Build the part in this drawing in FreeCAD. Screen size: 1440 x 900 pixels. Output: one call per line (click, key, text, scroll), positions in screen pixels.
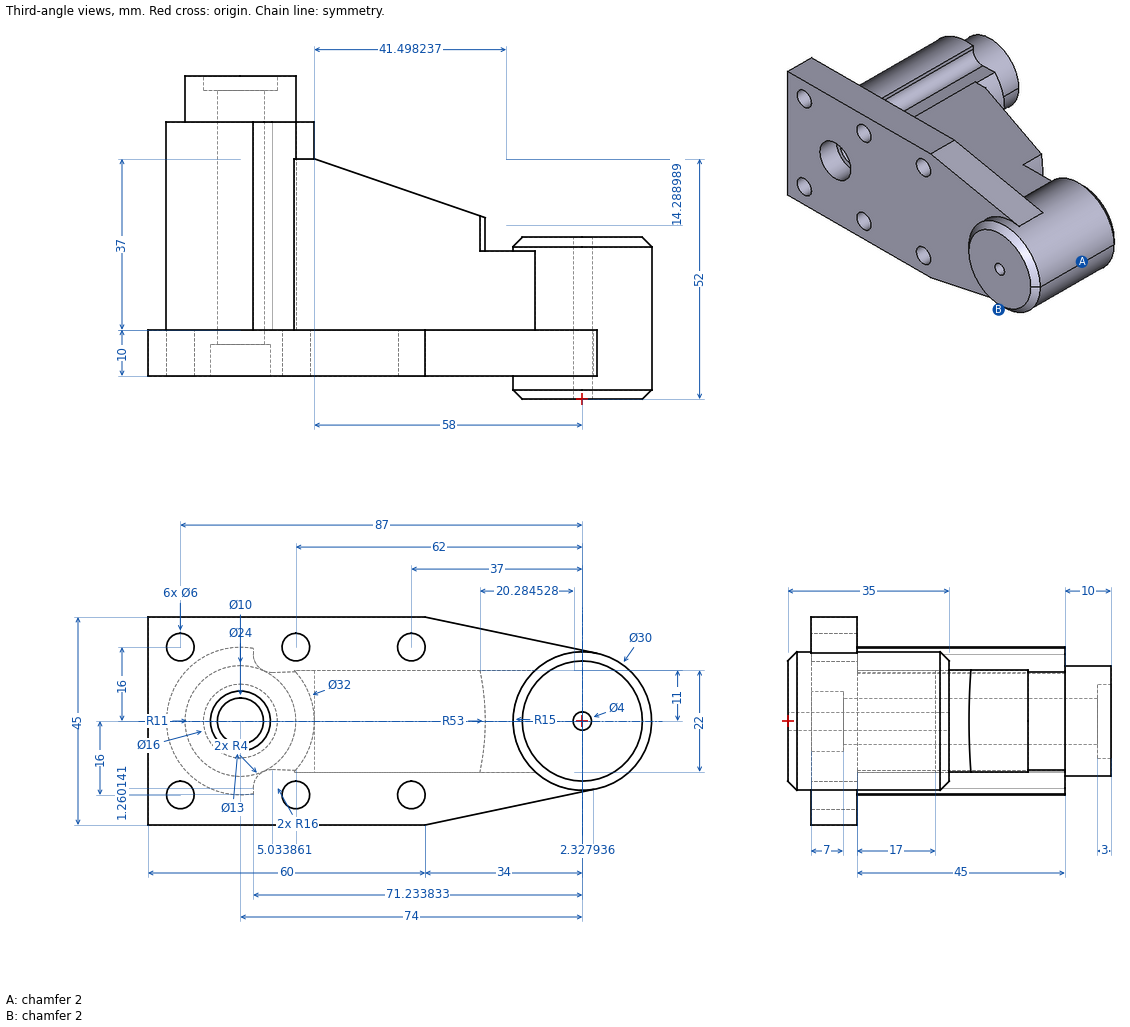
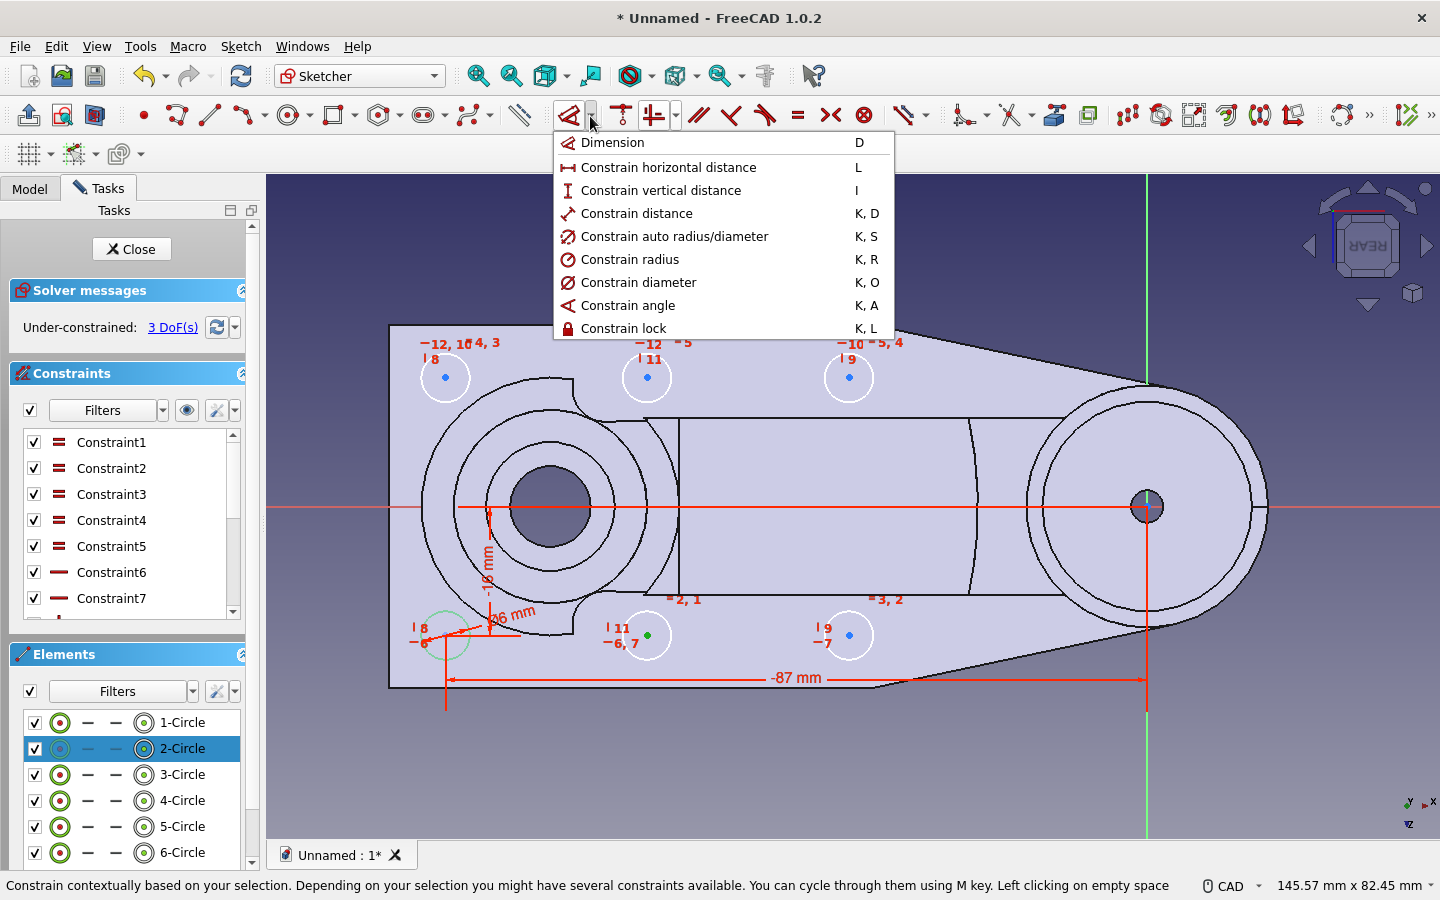
click(724, 168)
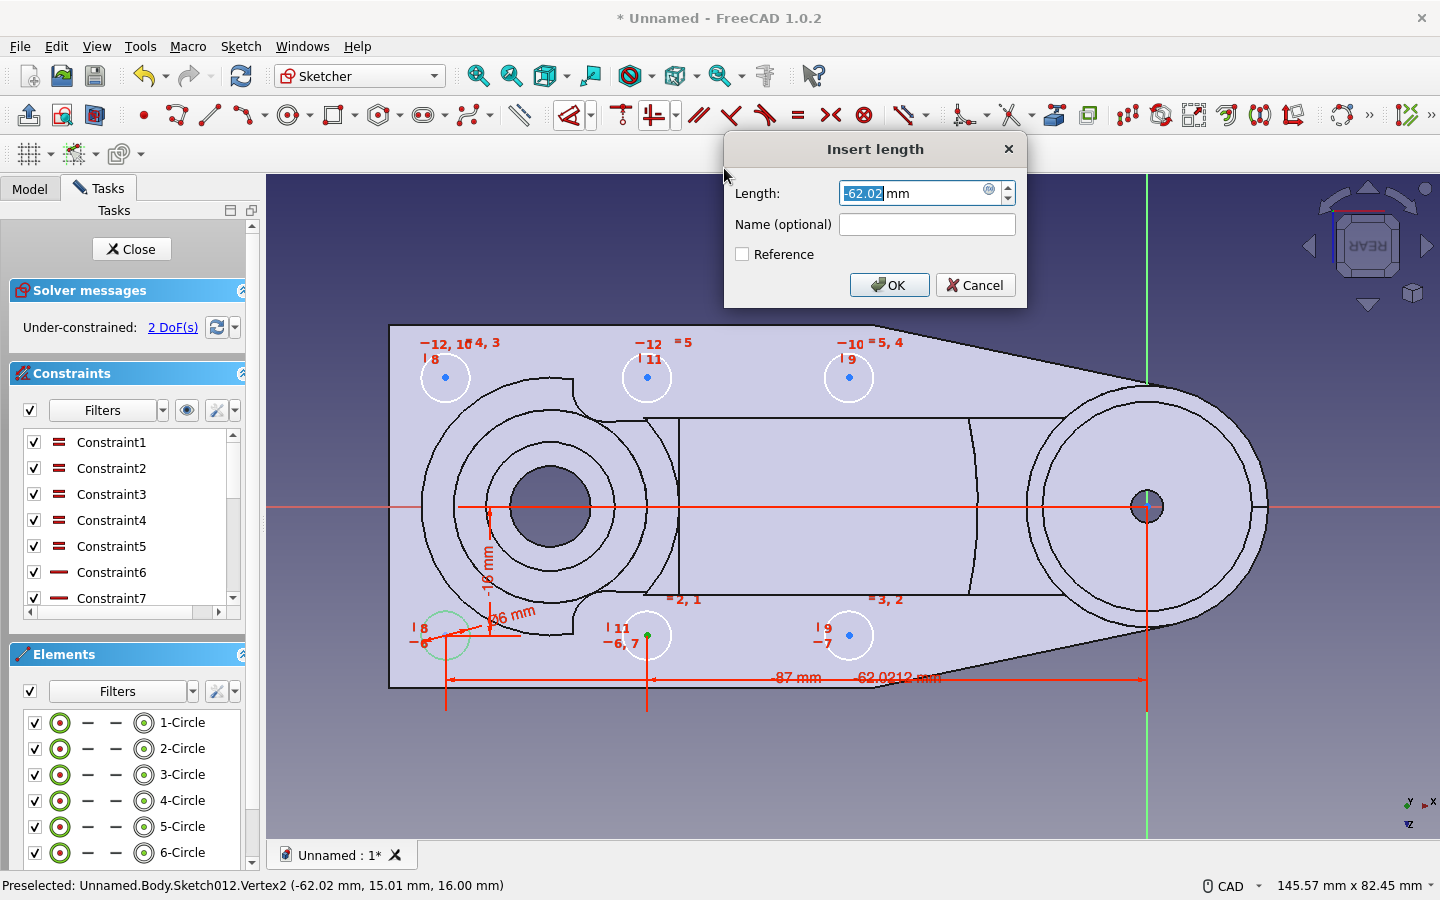
text(-62)
key(Return)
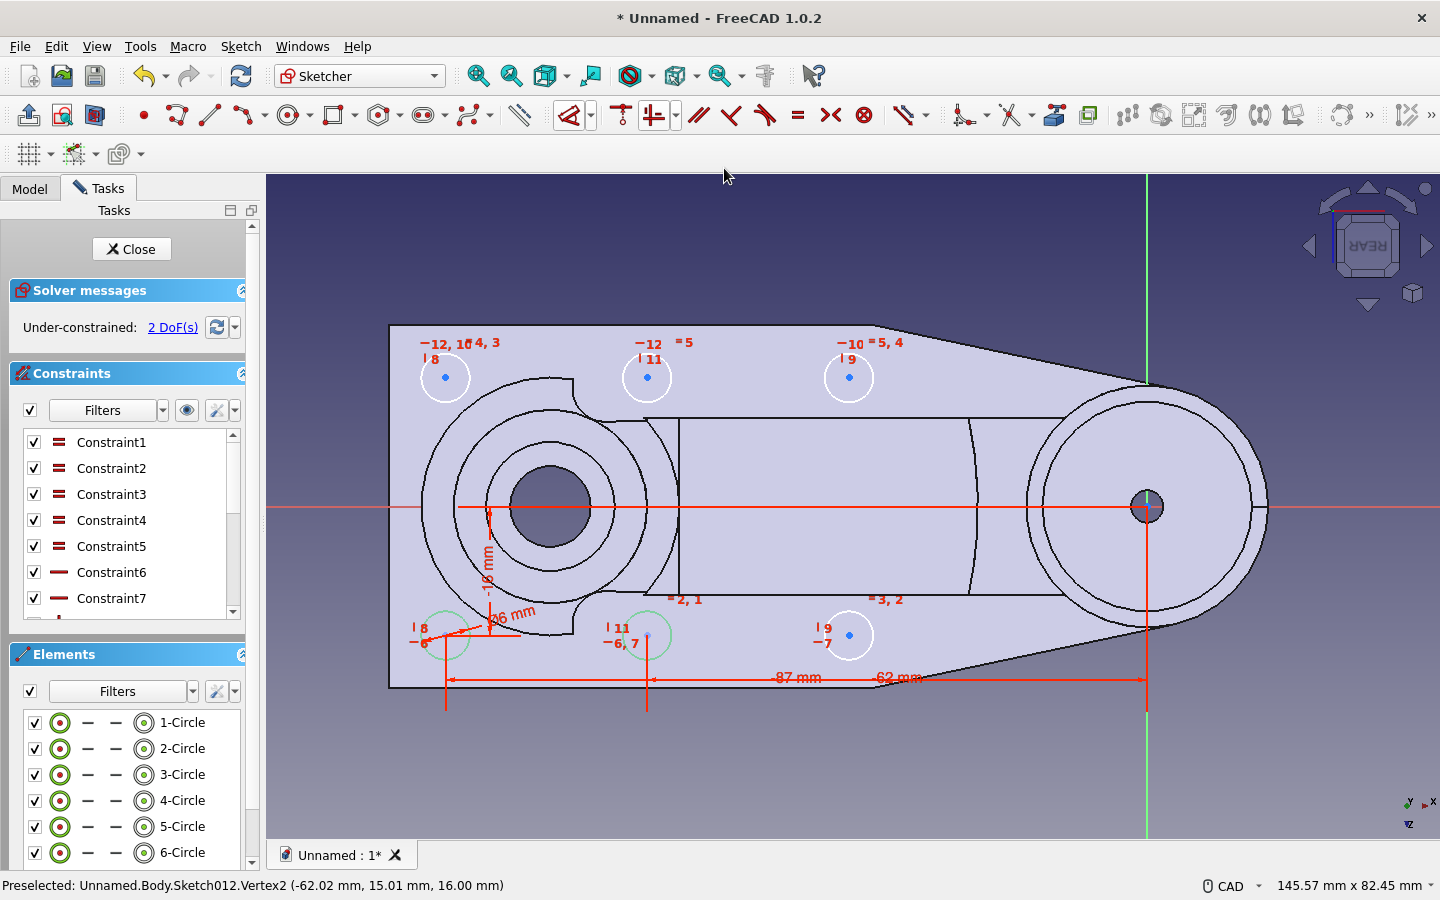
click(849, 636)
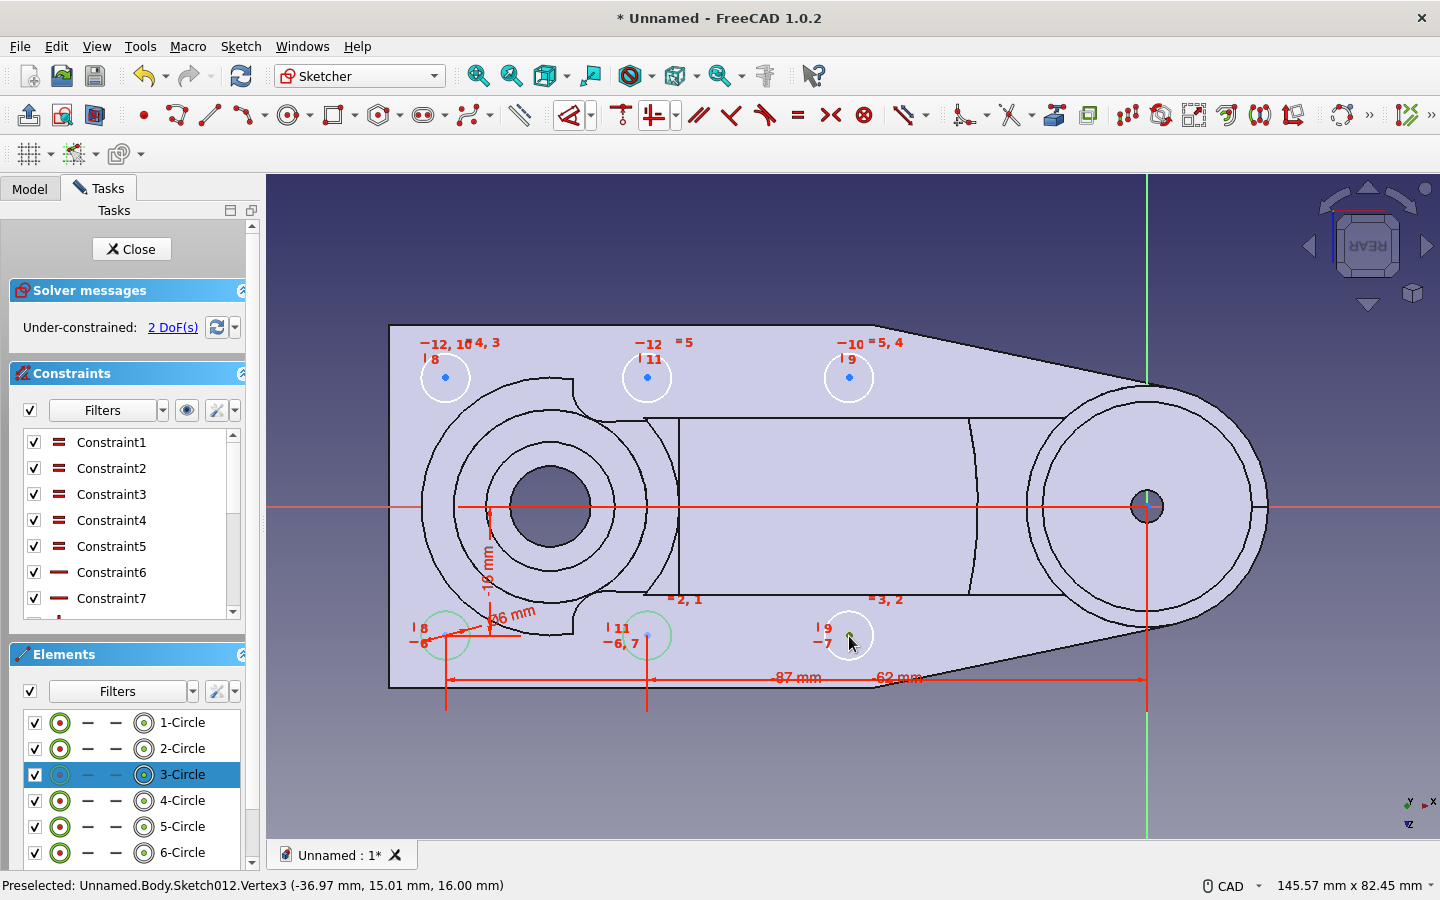
click(590, 116)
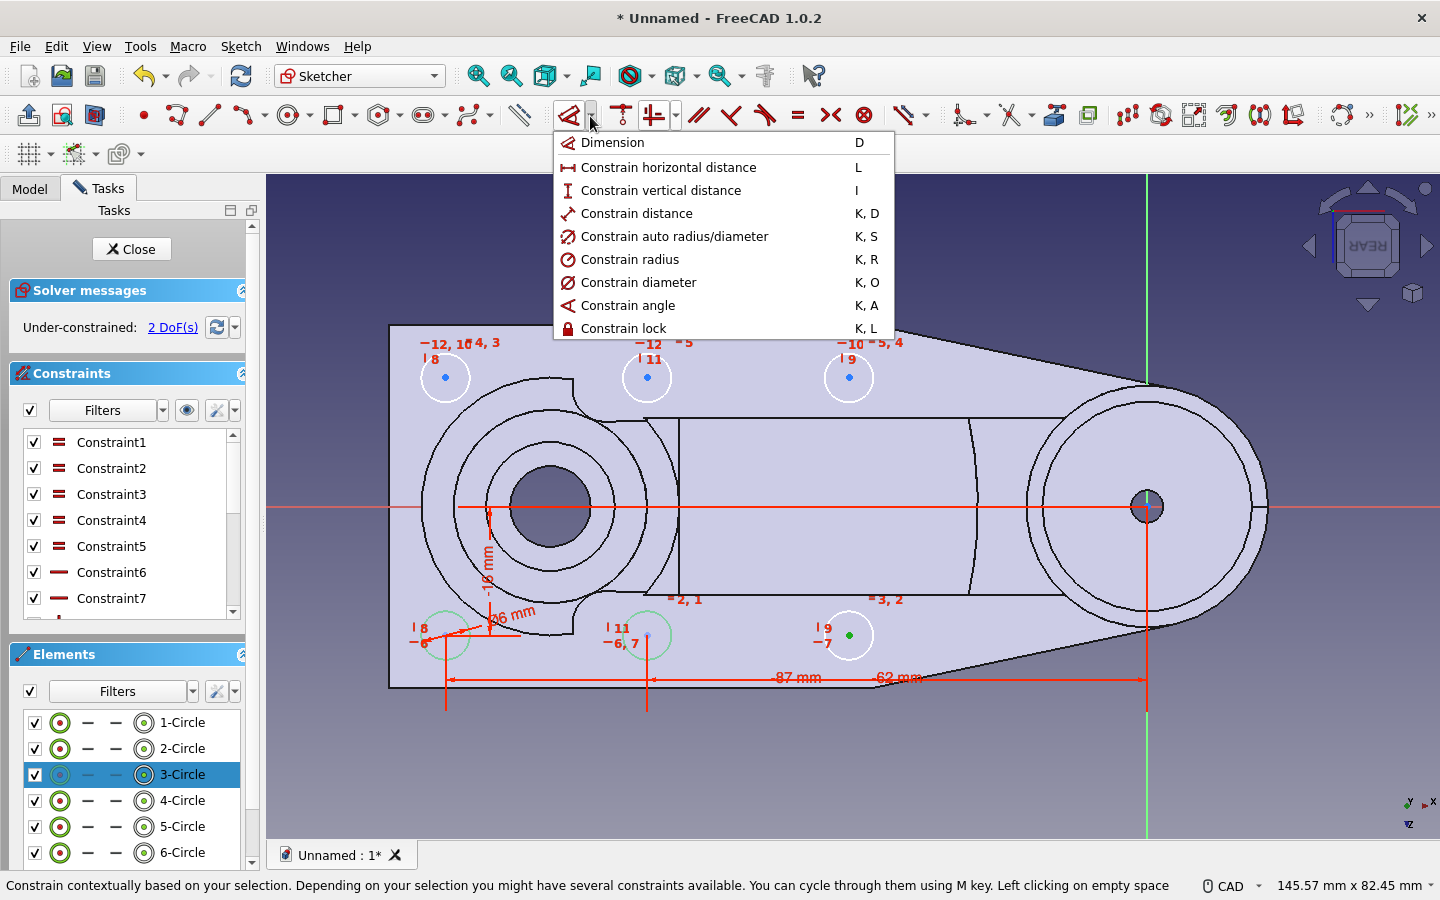
click(724, 168)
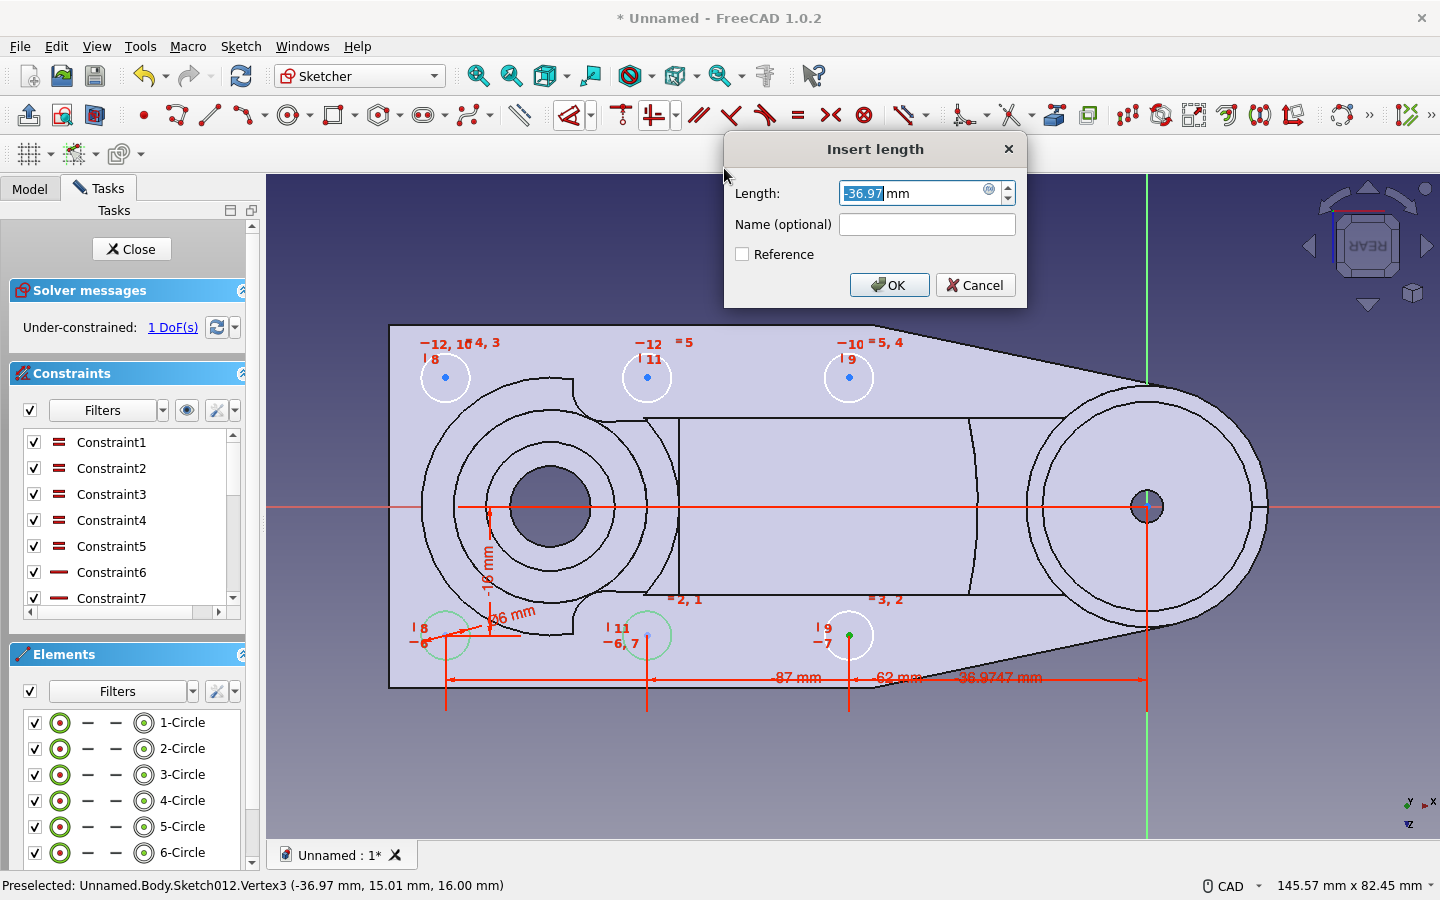
text(-37)
key(Return)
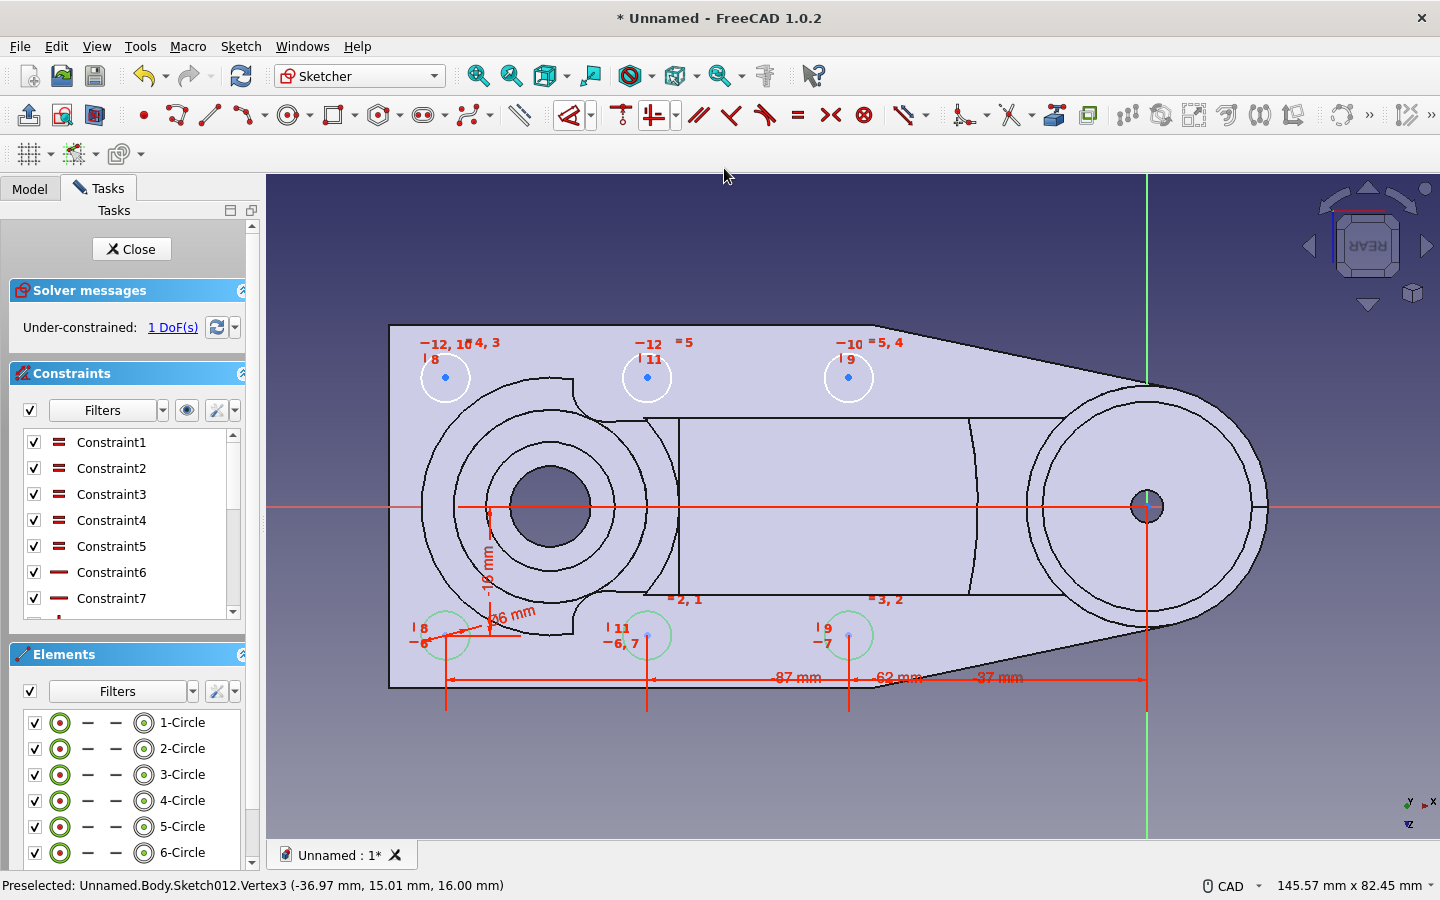
click(446, 378)